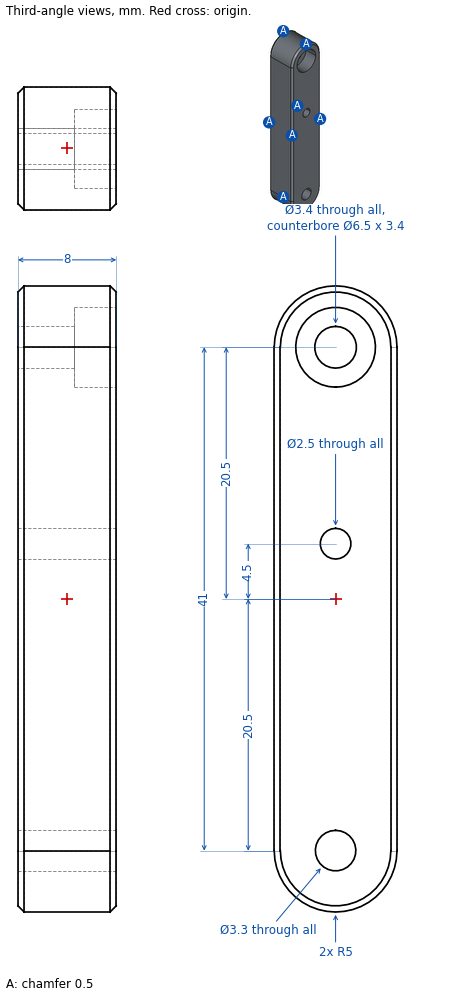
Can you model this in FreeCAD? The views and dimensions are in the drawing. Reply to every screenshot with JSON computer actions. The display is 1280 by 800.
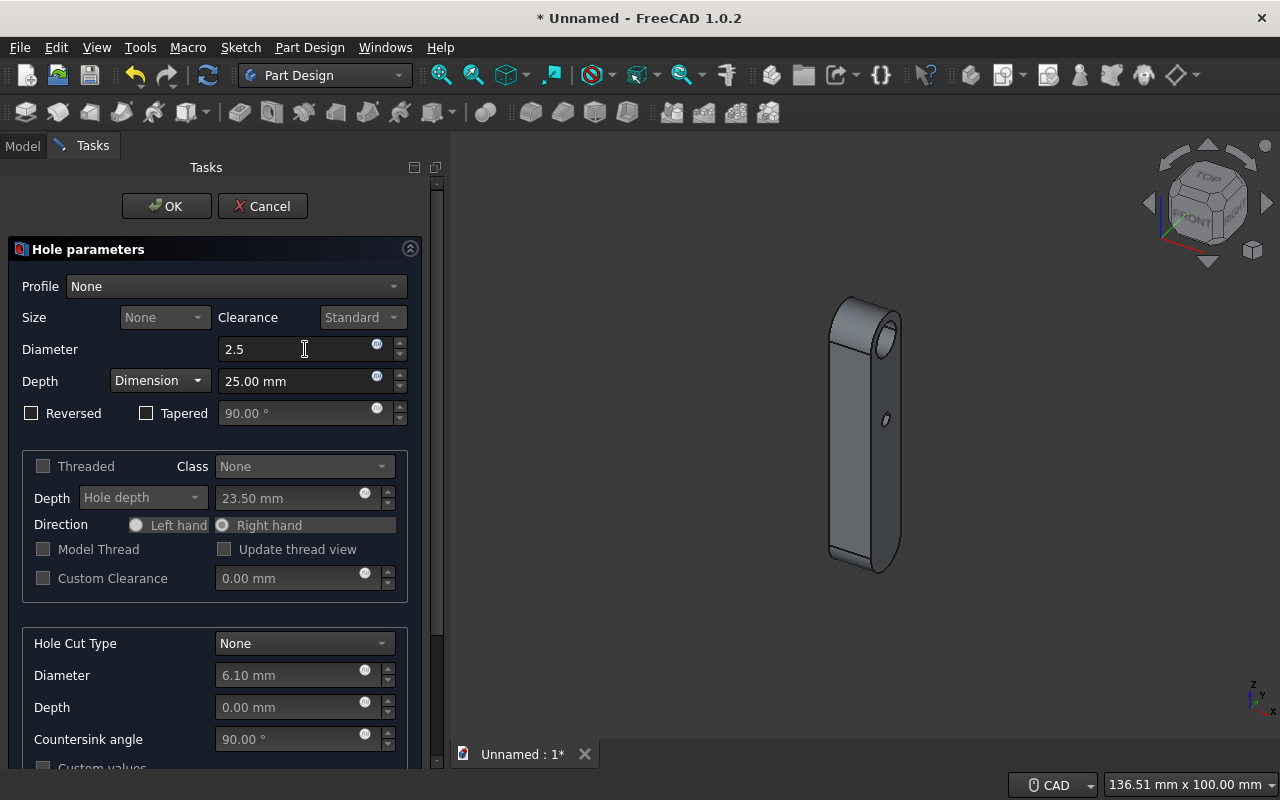
{"action": "left_click", "coordinate": [161, 380]}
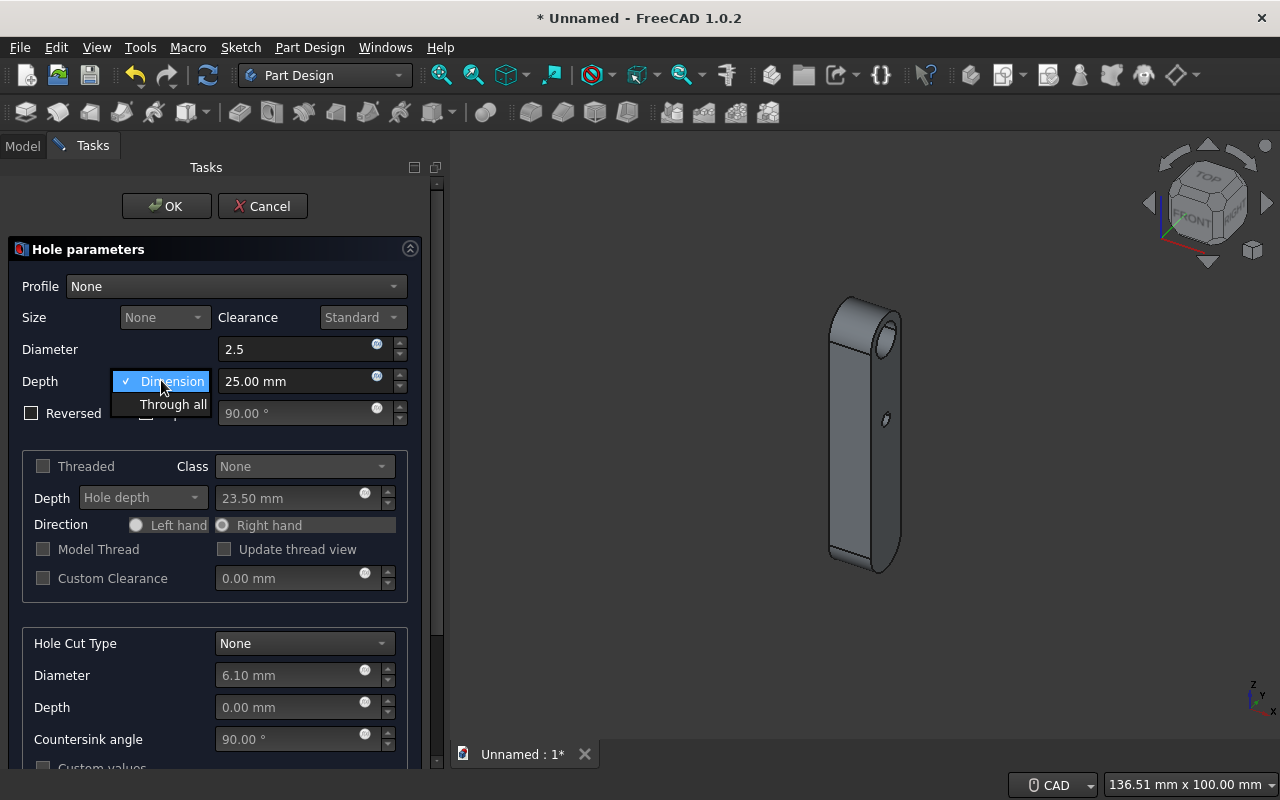
{"action": "left_click", "coordinate": [160, 404]}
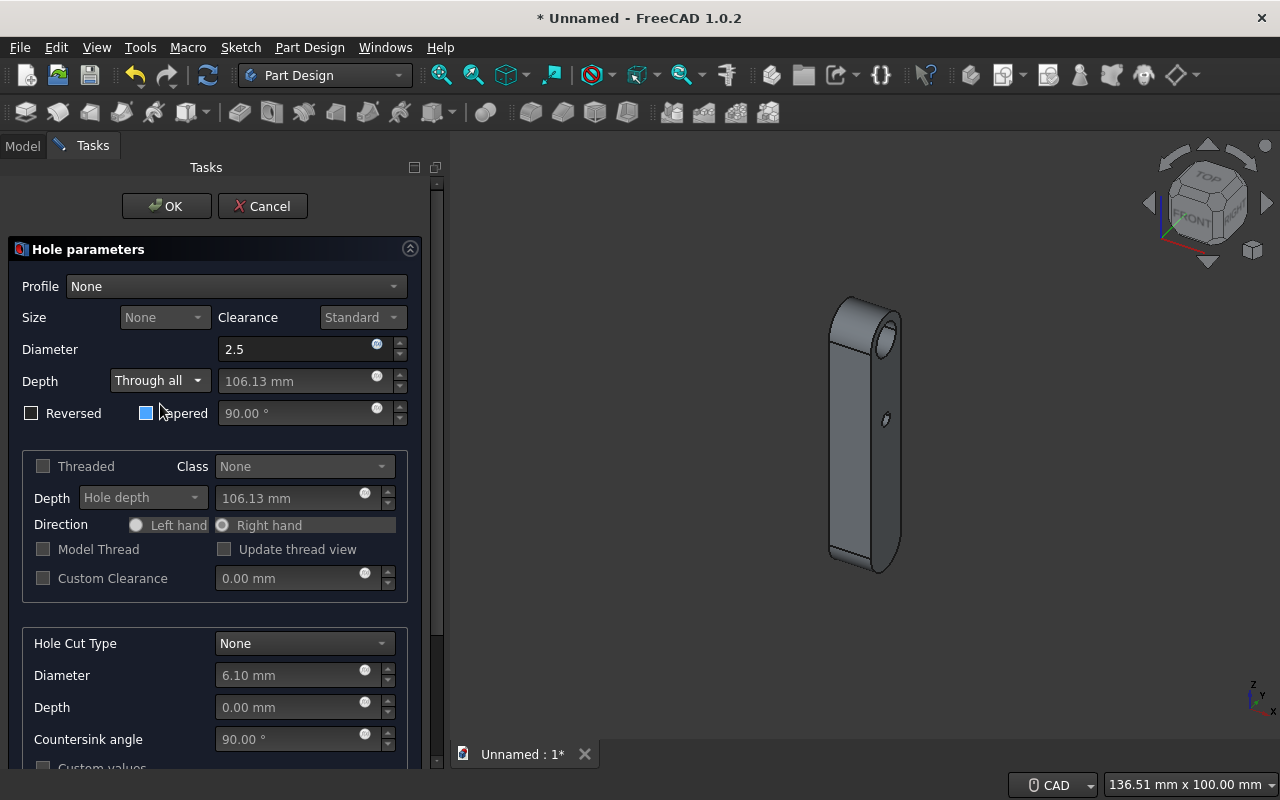
{"action": "left_click", "coordinate": [167, 206]}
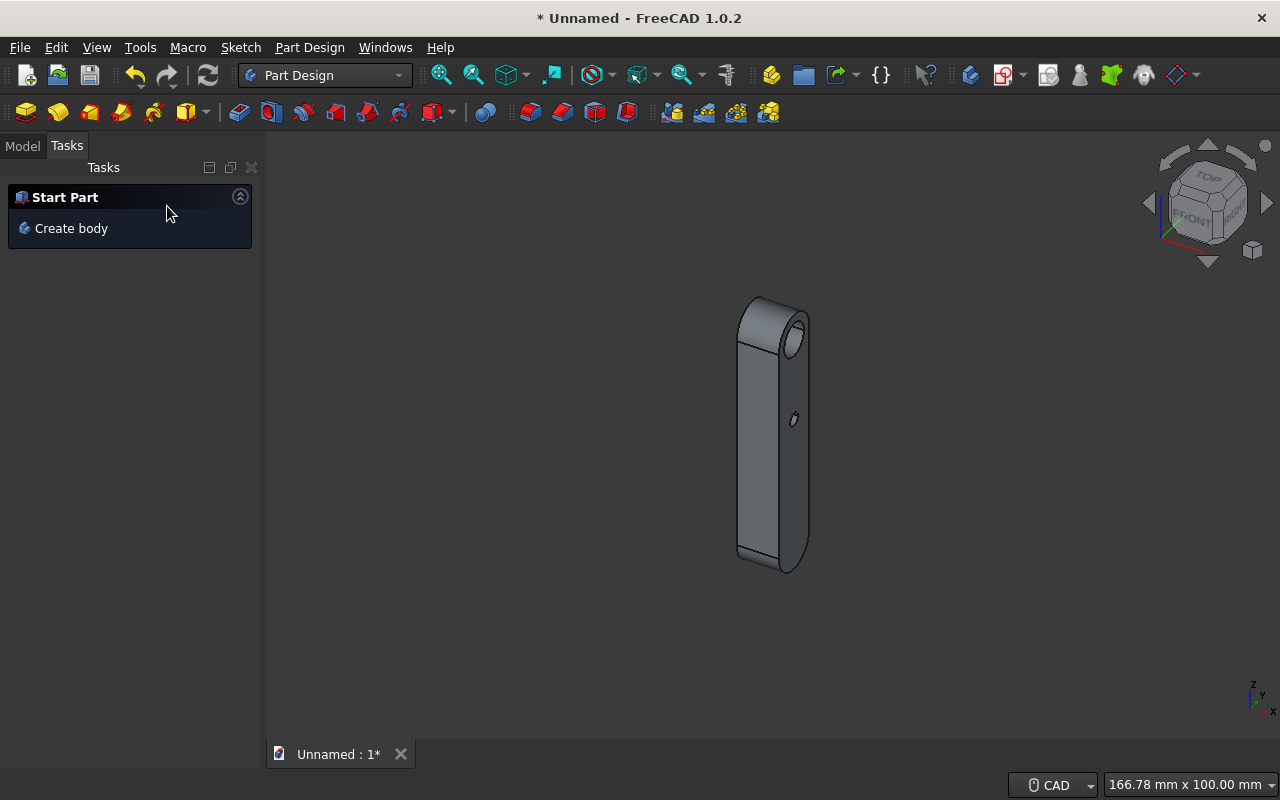
{"action": "left_click", "coordinate": [794, 477]}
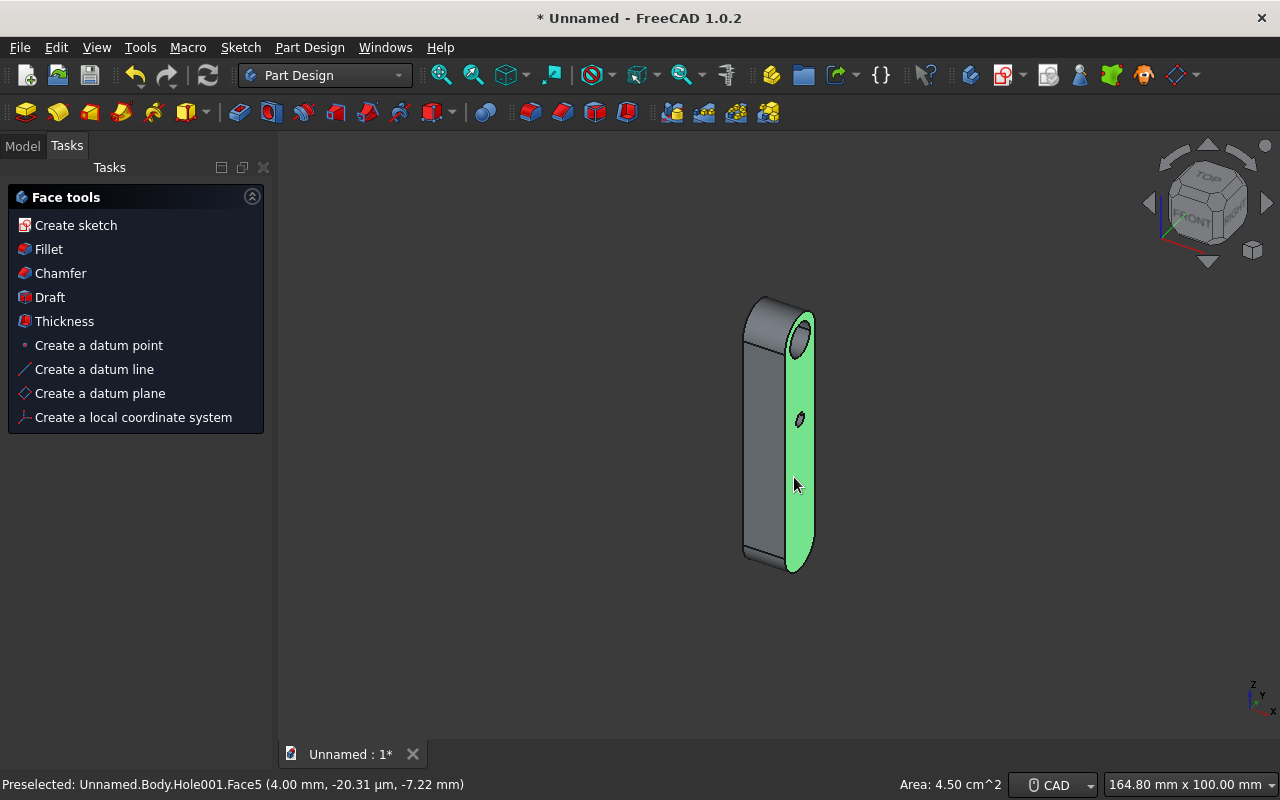
{"action": "left_click", "coordinate": [1004, 76]}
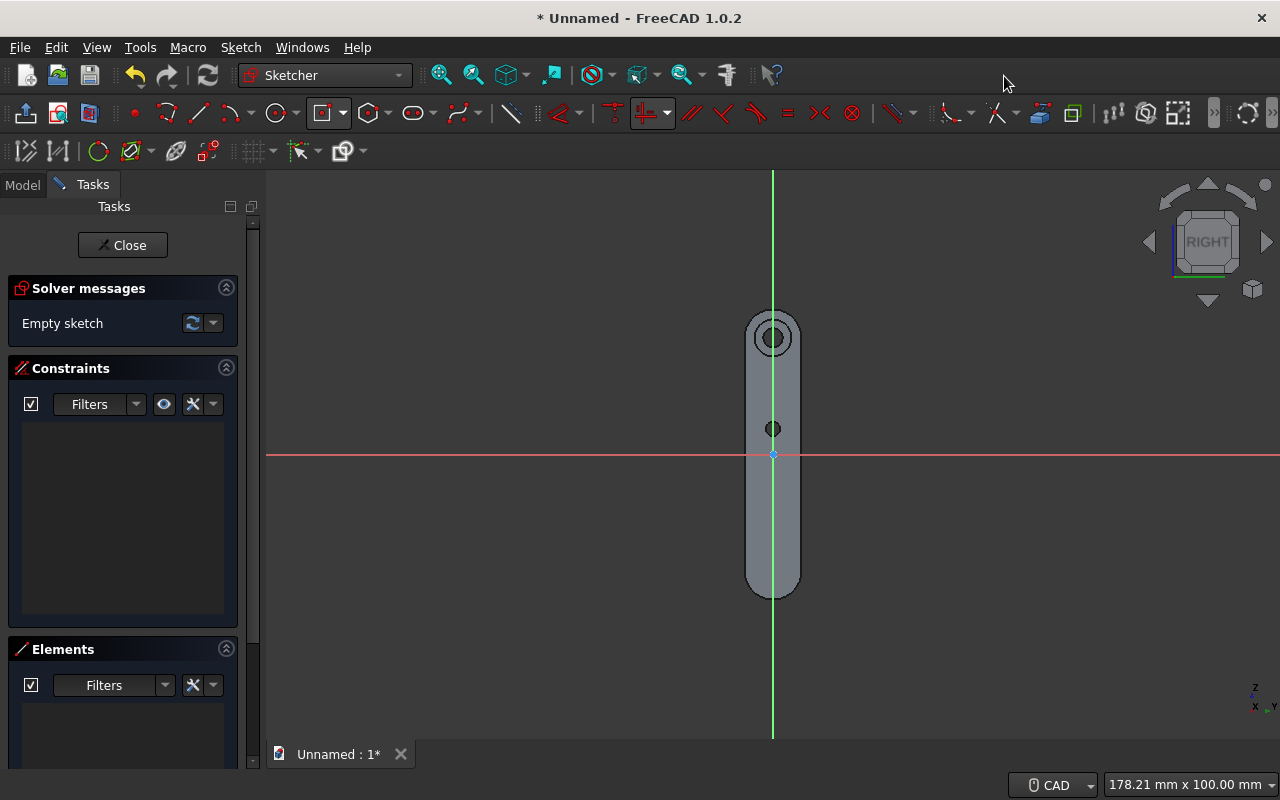
{"action": "scroll", "coordinate": [777, 577], "scroll_direction": "up", "scroll_amount": 15}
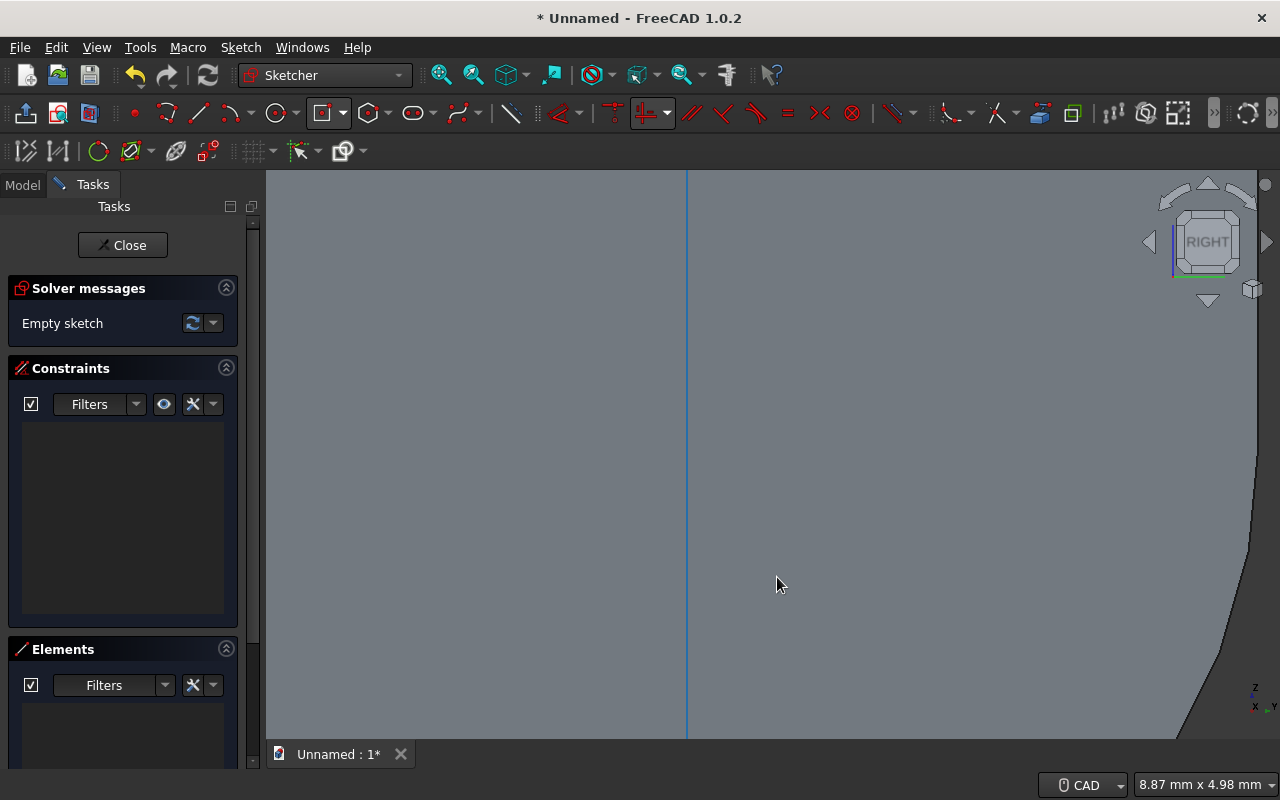
{"action": "key", "text": "g c"}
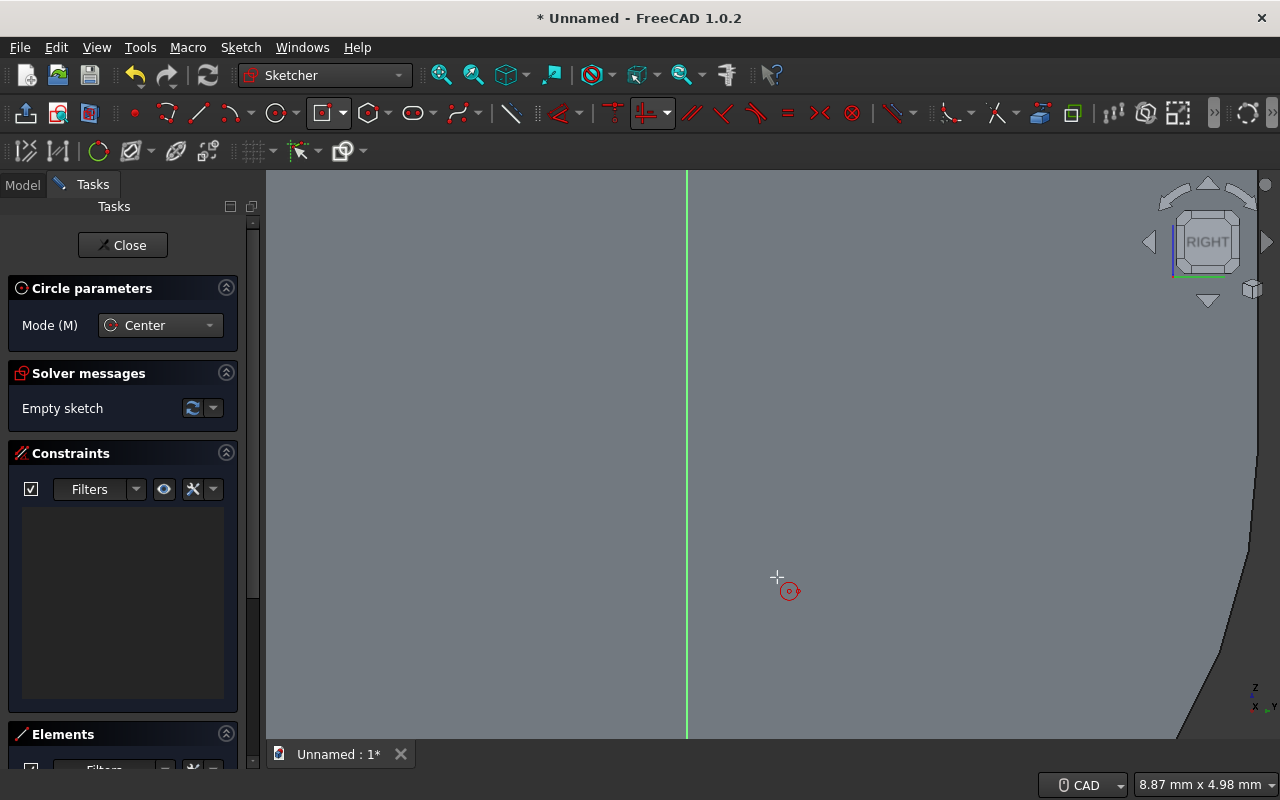
{"action": "left_click", "coordinate": [687, 446]}
{"action": "left_click", "coordinate": [820, 312]}
{"action": "key", "text": "Escape"}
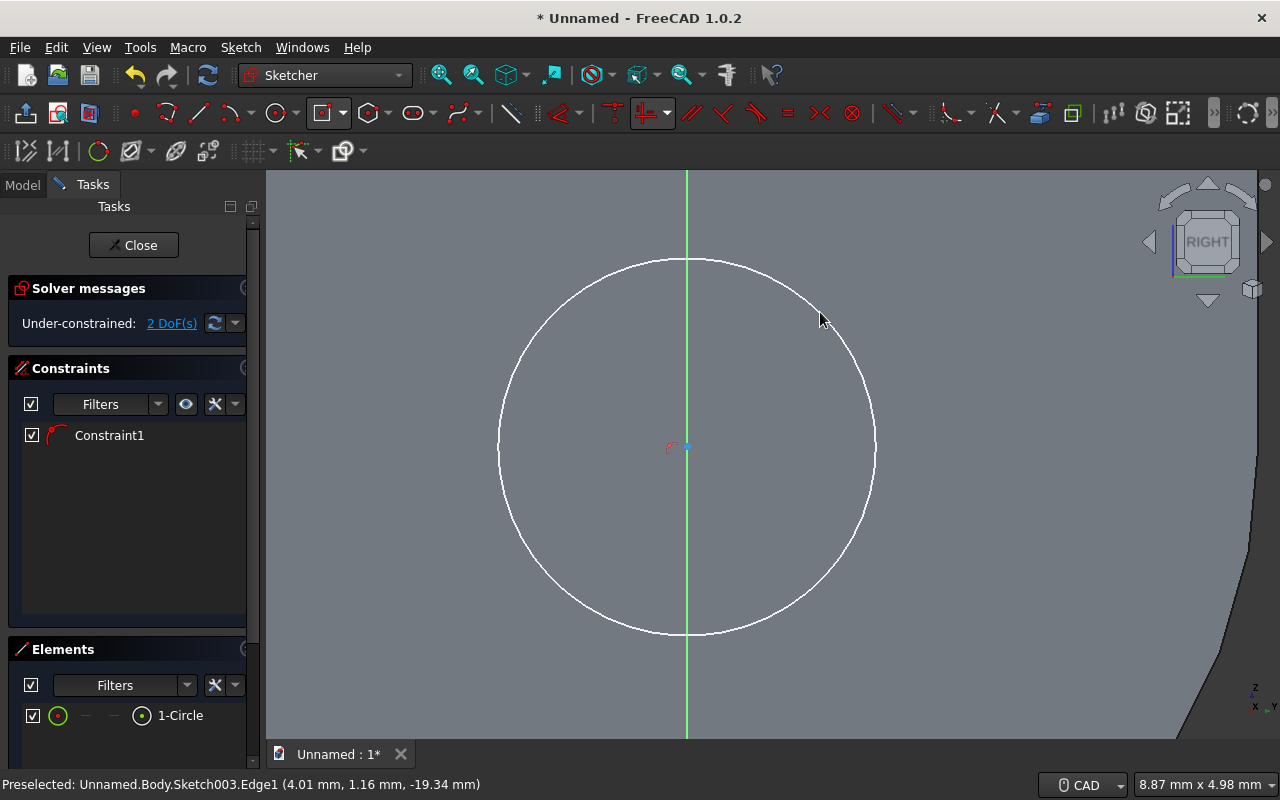
{"action": "key", "text": "d"}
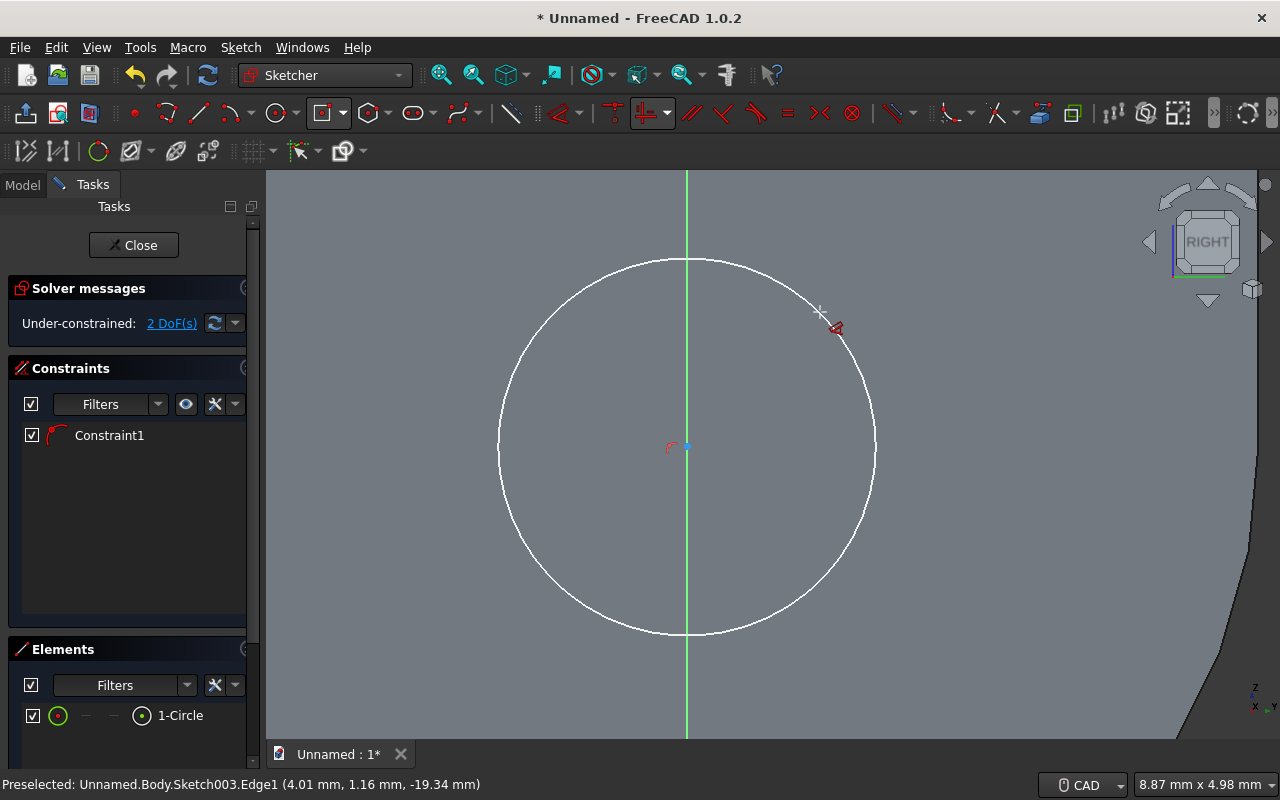
{"action": "left_click", "coordinate": [820, 313]}
{"action": "left_click", "coordinate": [843, 290]}